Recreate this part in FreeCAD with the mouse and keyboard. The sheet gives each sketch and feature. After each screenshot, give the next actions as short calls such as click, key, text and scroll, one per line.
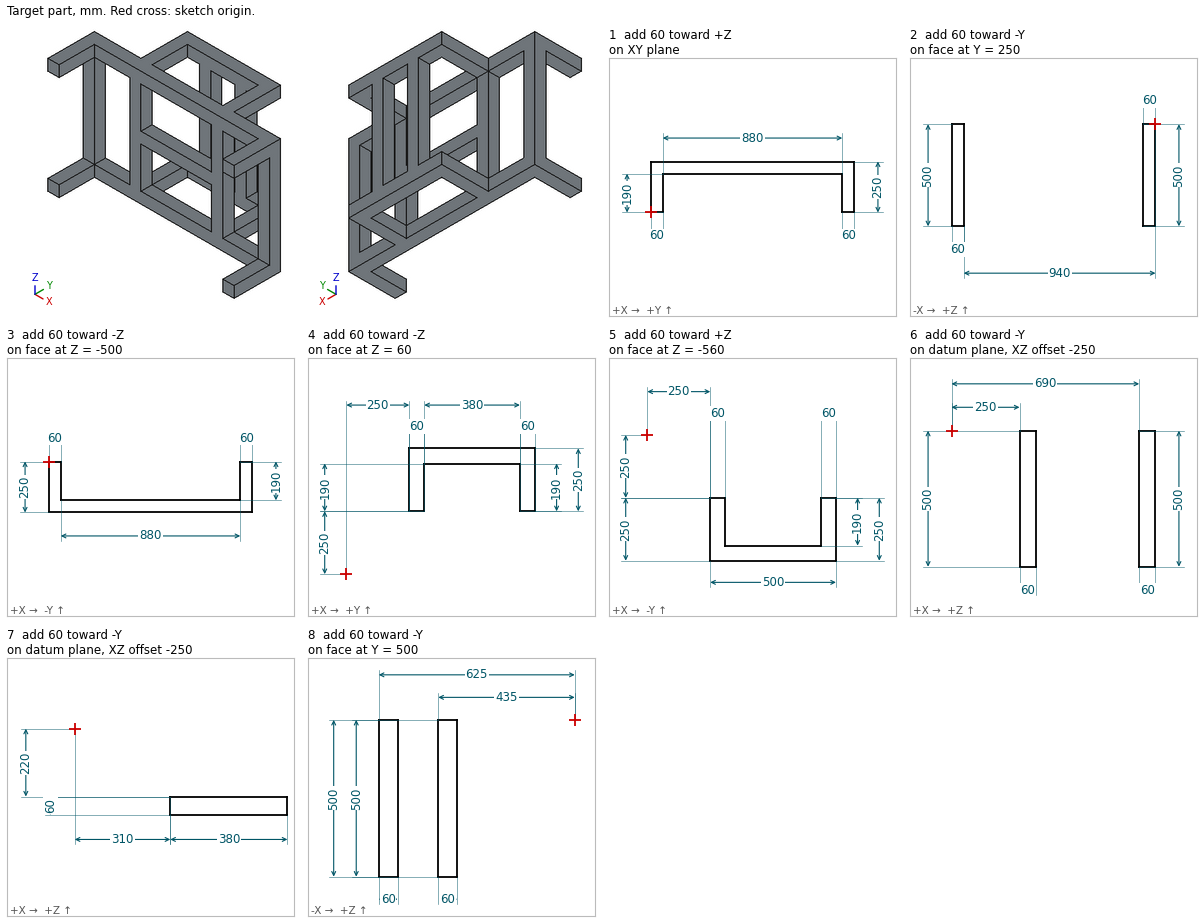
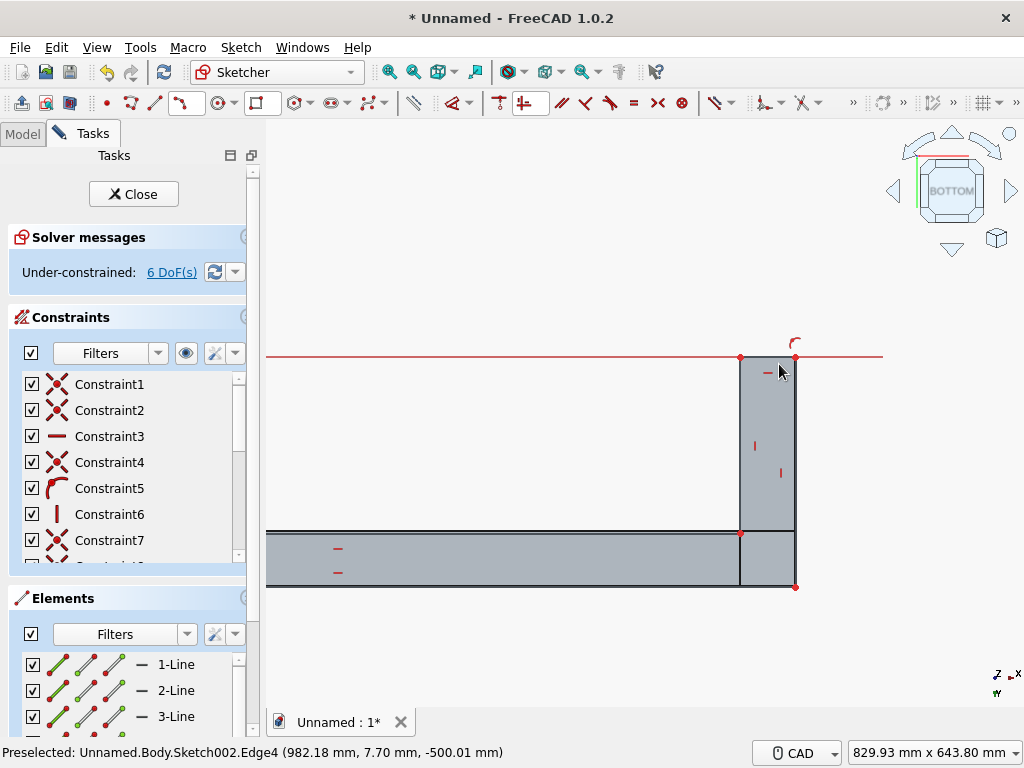
scroll(771, 365, down, 4)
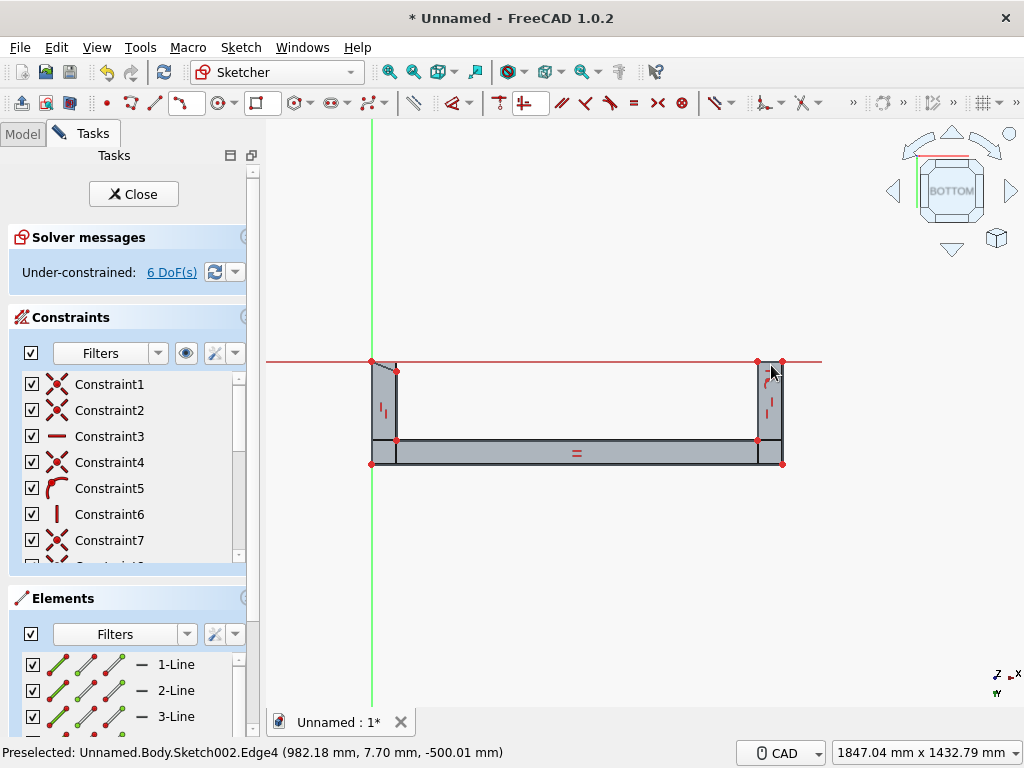
scroll(389, 369, up, 4)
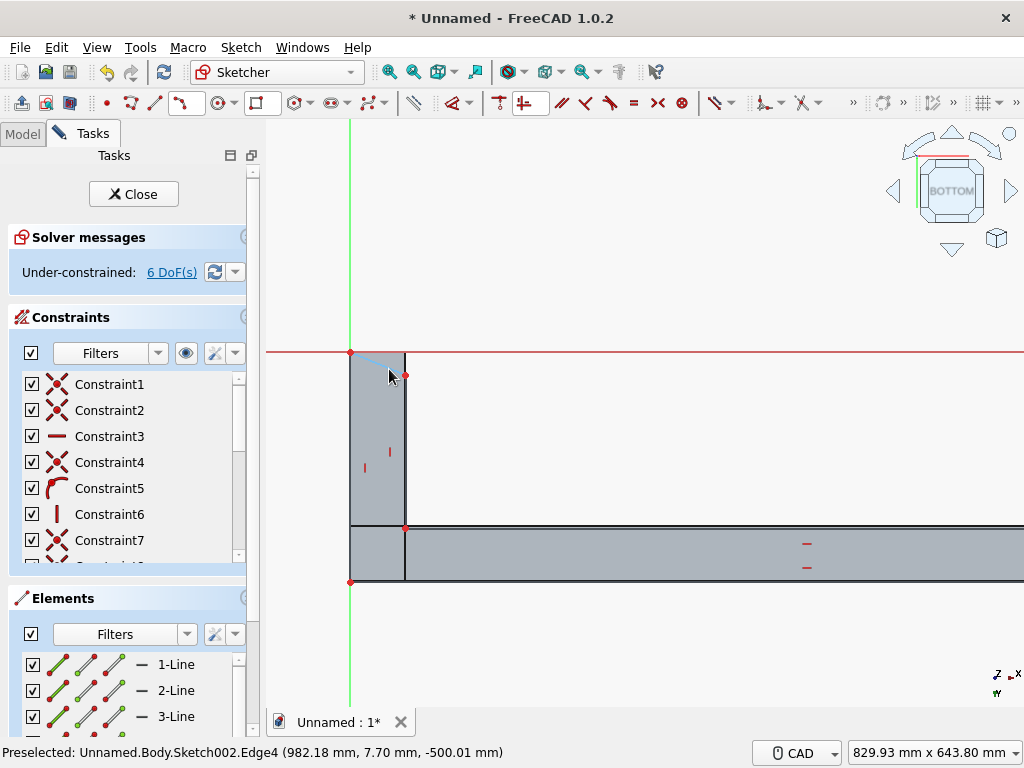
click(389, 368)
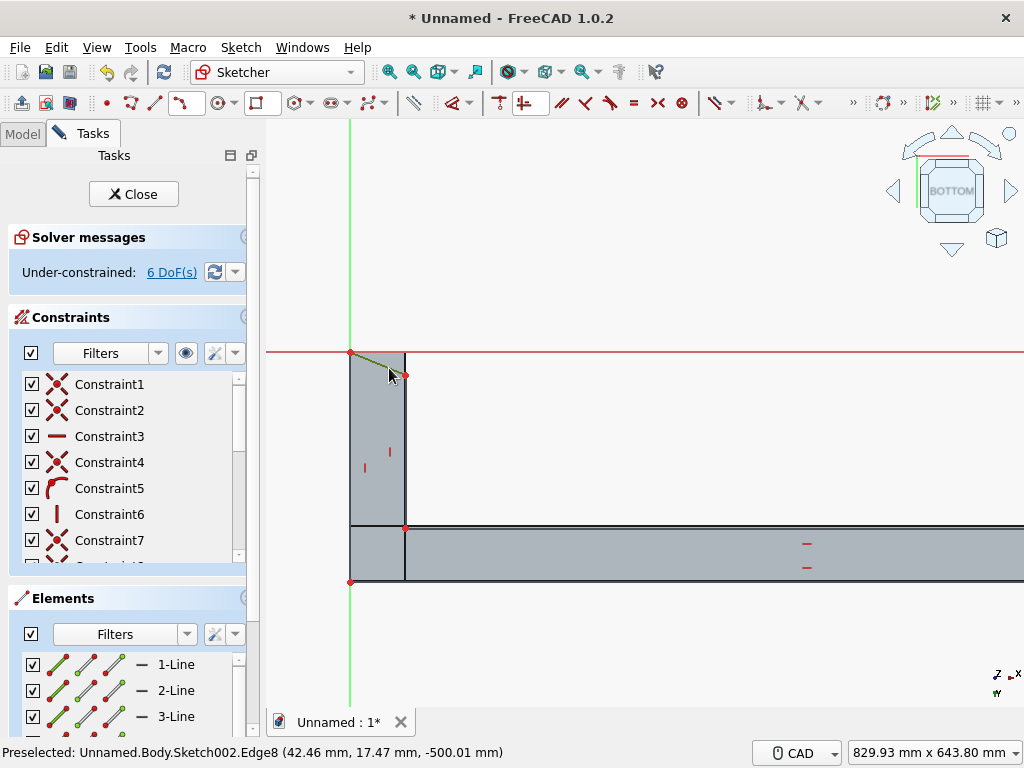
key(h)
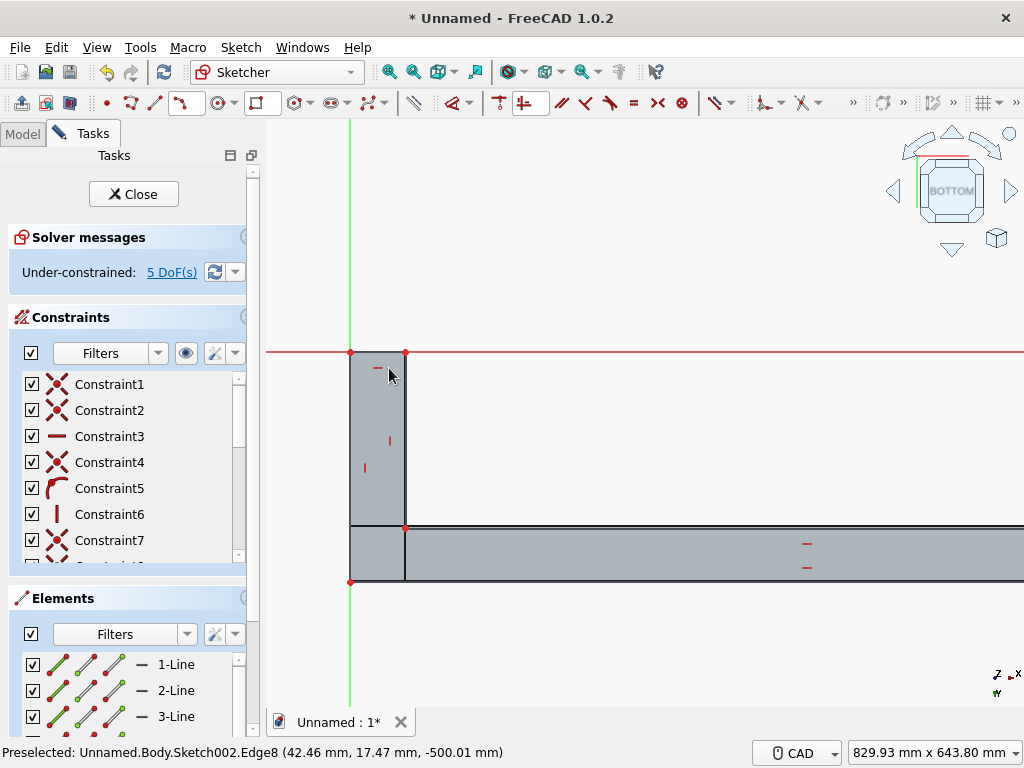
click(452, 104)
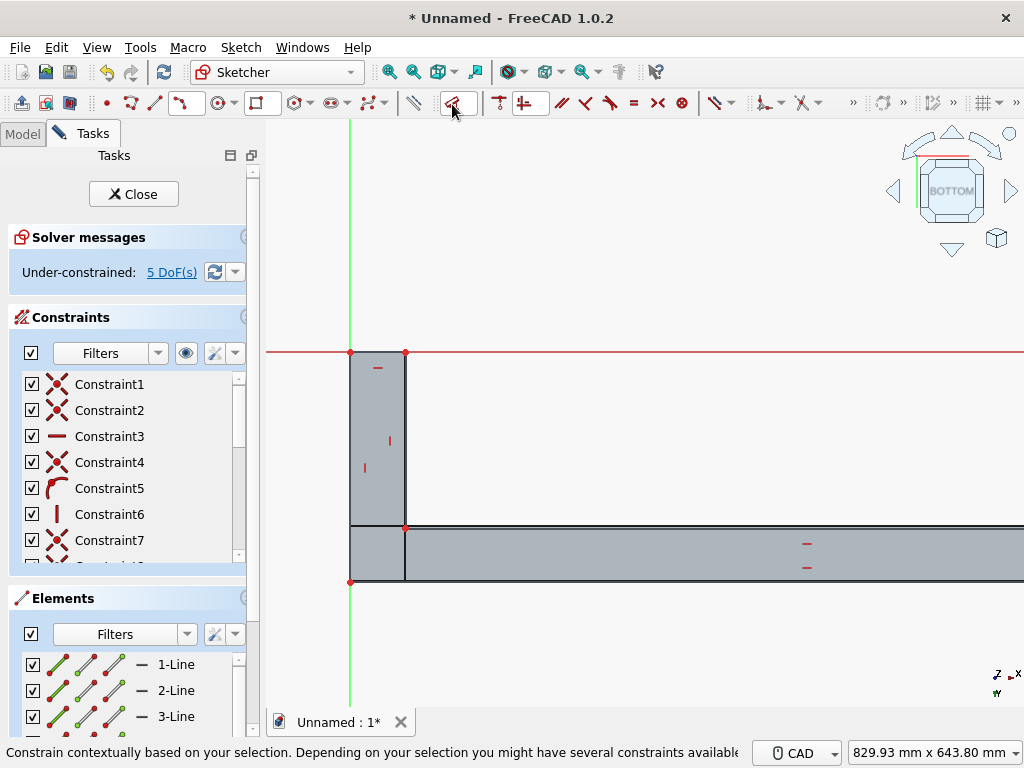
scroll(388, 369, down, 4)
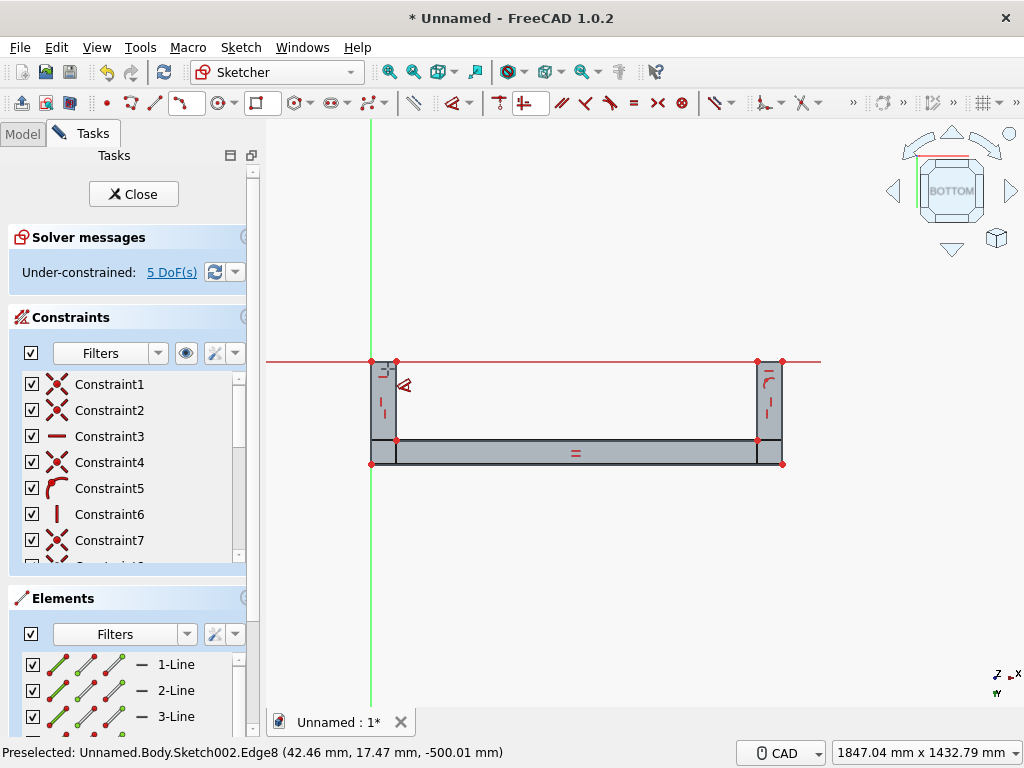
scroll(775, 362, up, 4)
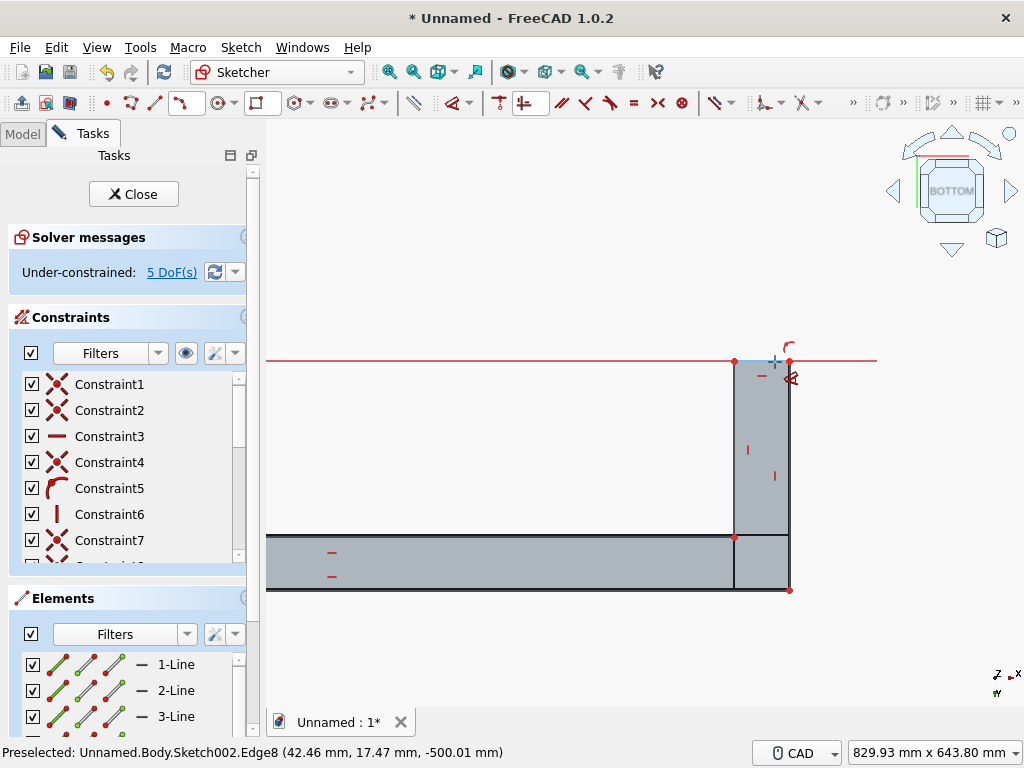
click(773, 361)
click(762, 327)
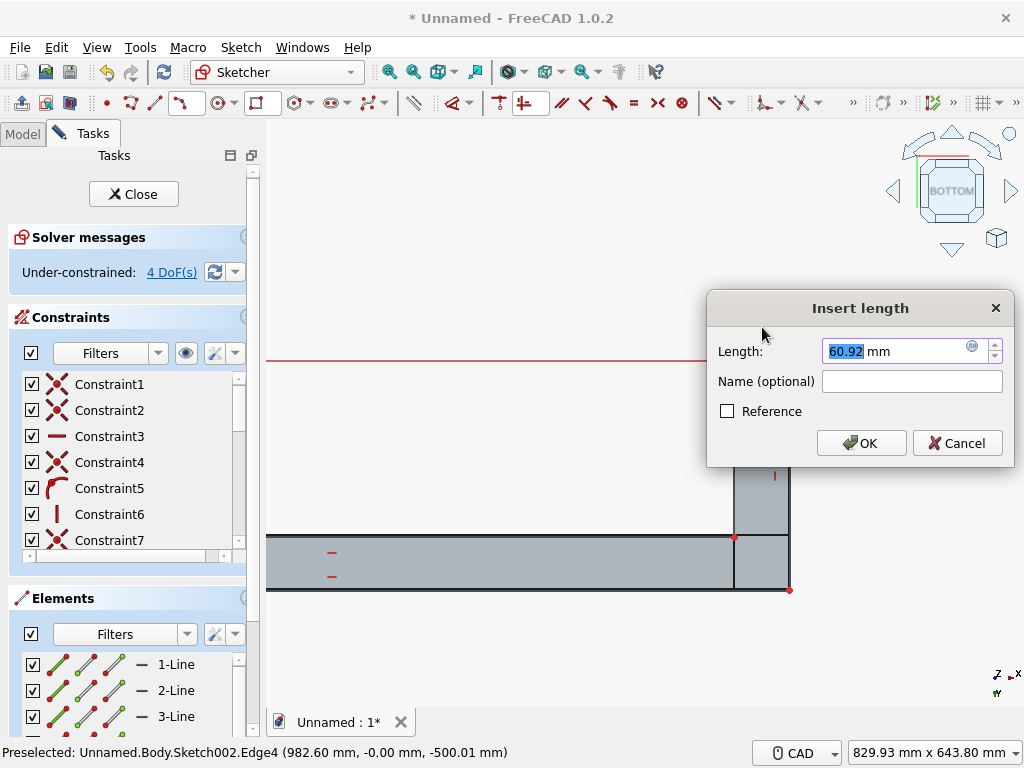
text(60)
key(Return)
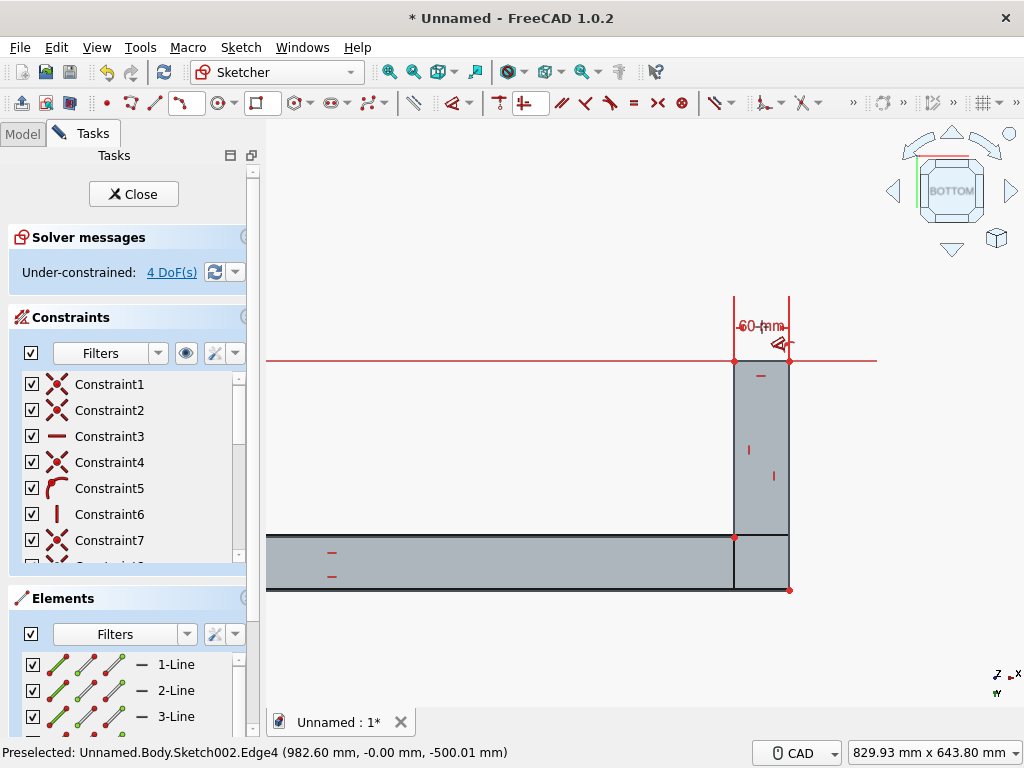
scroll(776, 362, down, 4)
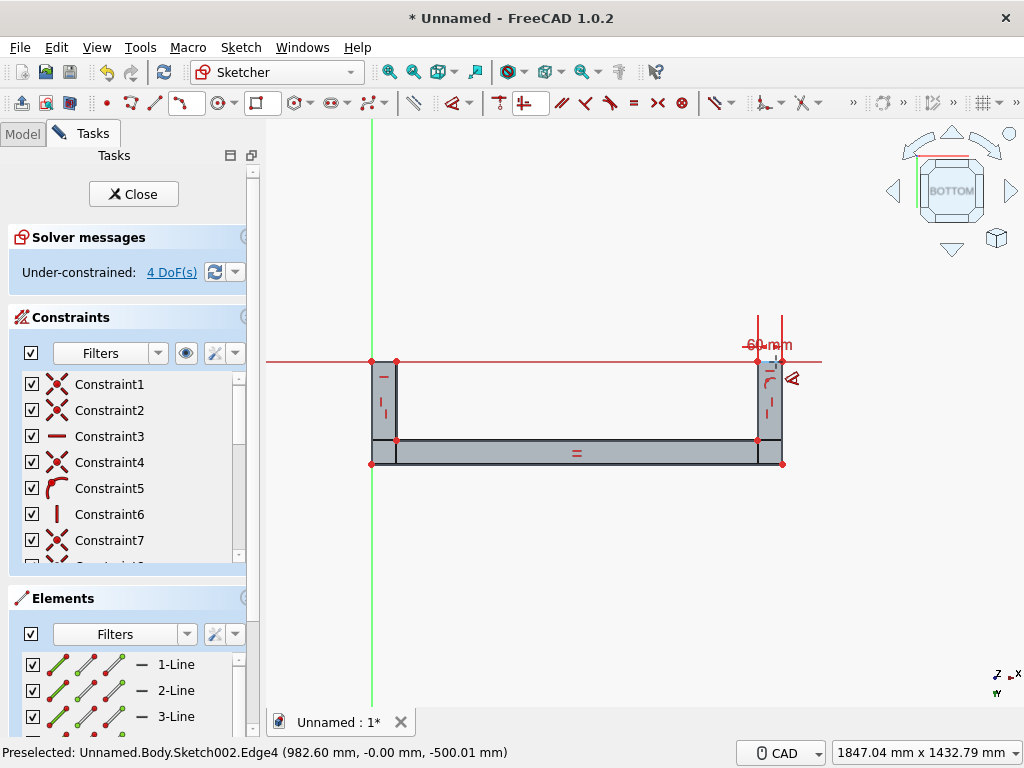
scroll(389, 362, up, 4)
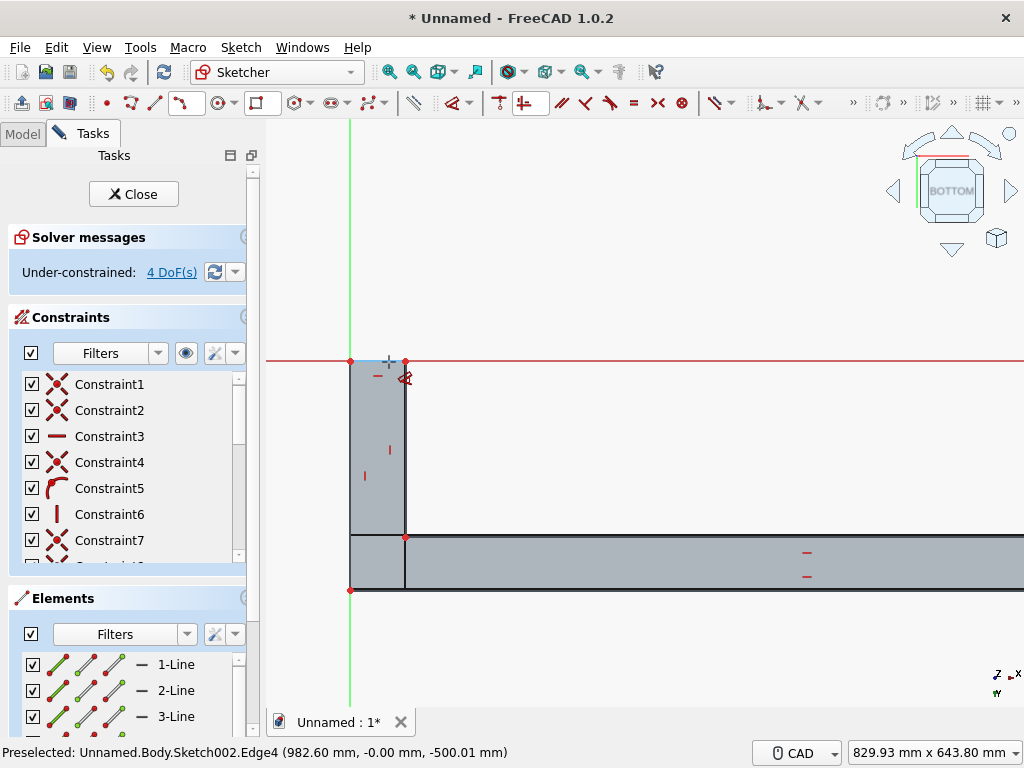
click(389, 361)
click(378, 327)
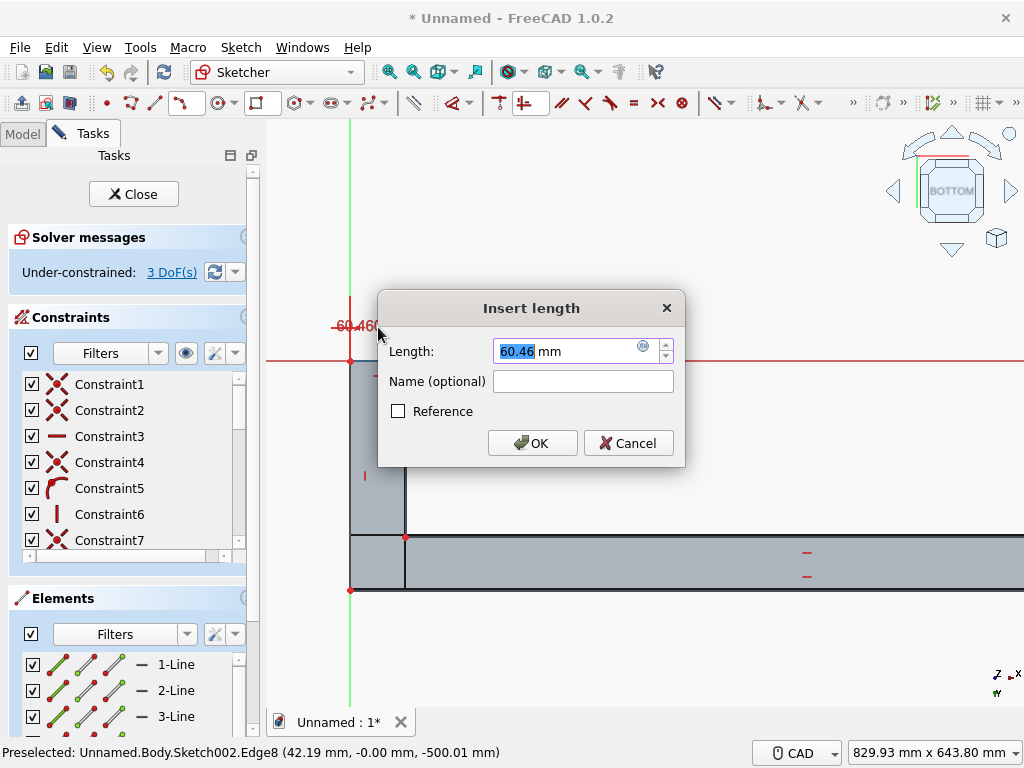
text(60)
key(Return)